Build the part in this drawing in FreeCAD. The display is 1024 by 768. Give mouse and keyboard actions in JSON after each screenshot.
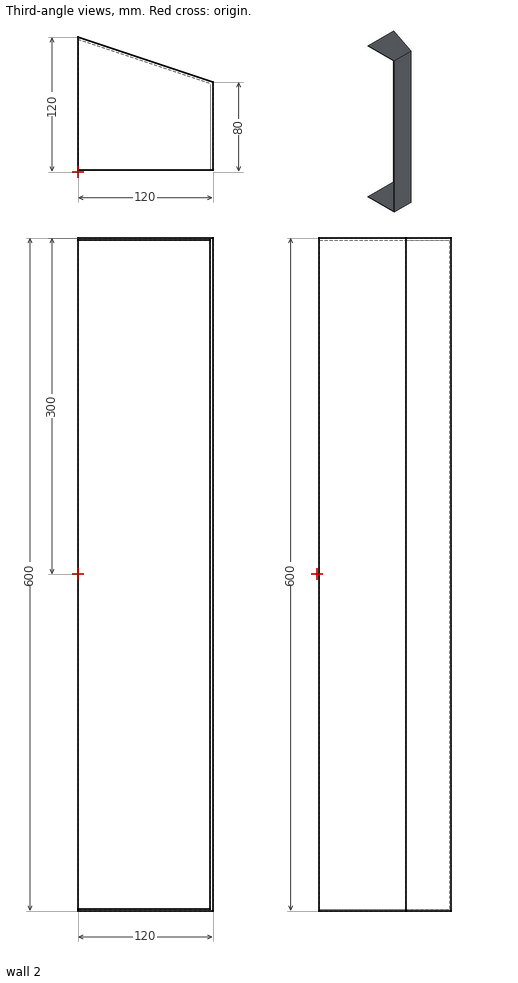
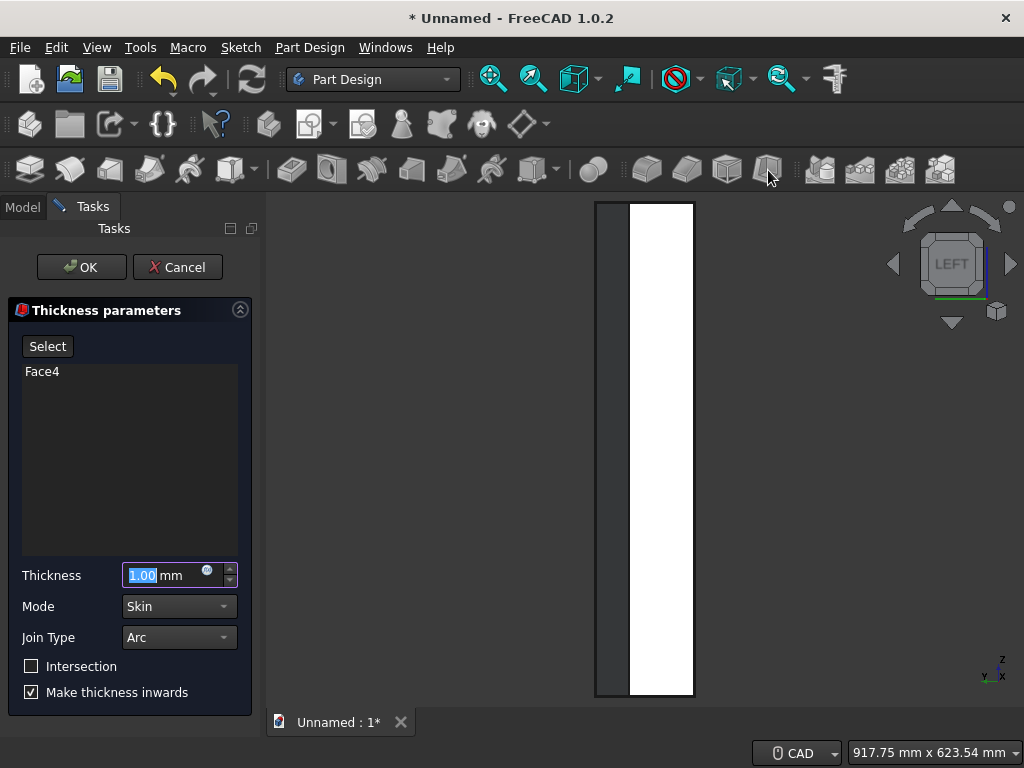
{"action": "type", "text": "2"}
{"action": "key", "text": "Tab"}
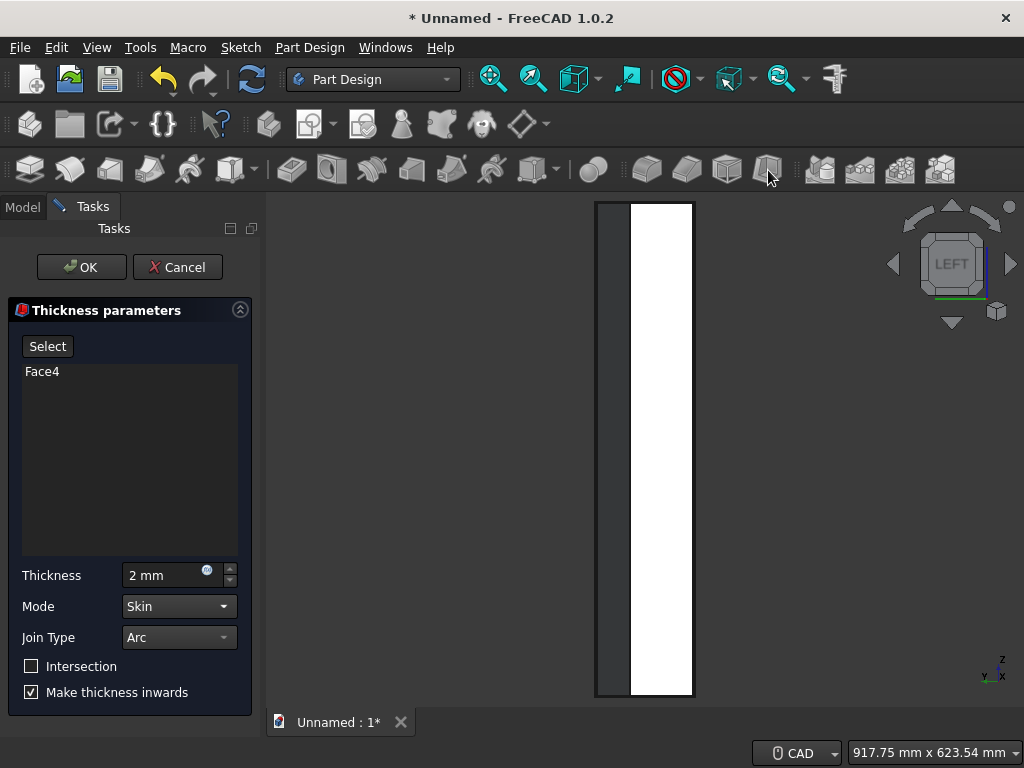
{"action": "left_click", "coordinate": [180, 638]}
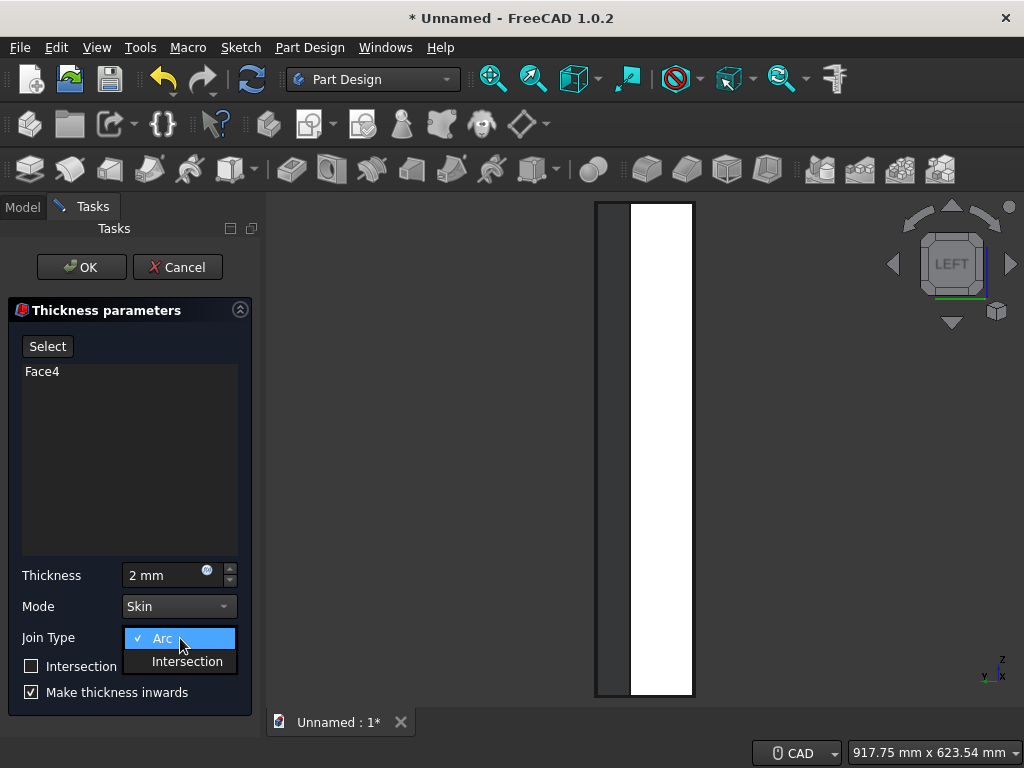
{"action": "left_click", "coordinate": [179, 662]}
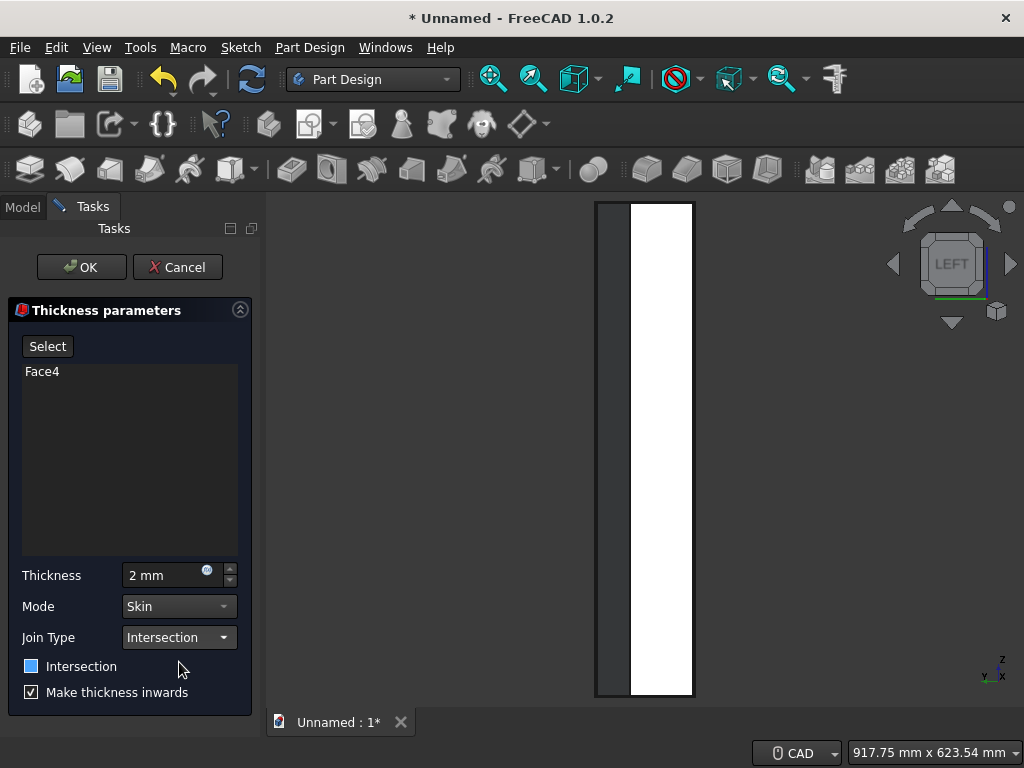
{"action": "left_click", "coordinate": [82, 267]}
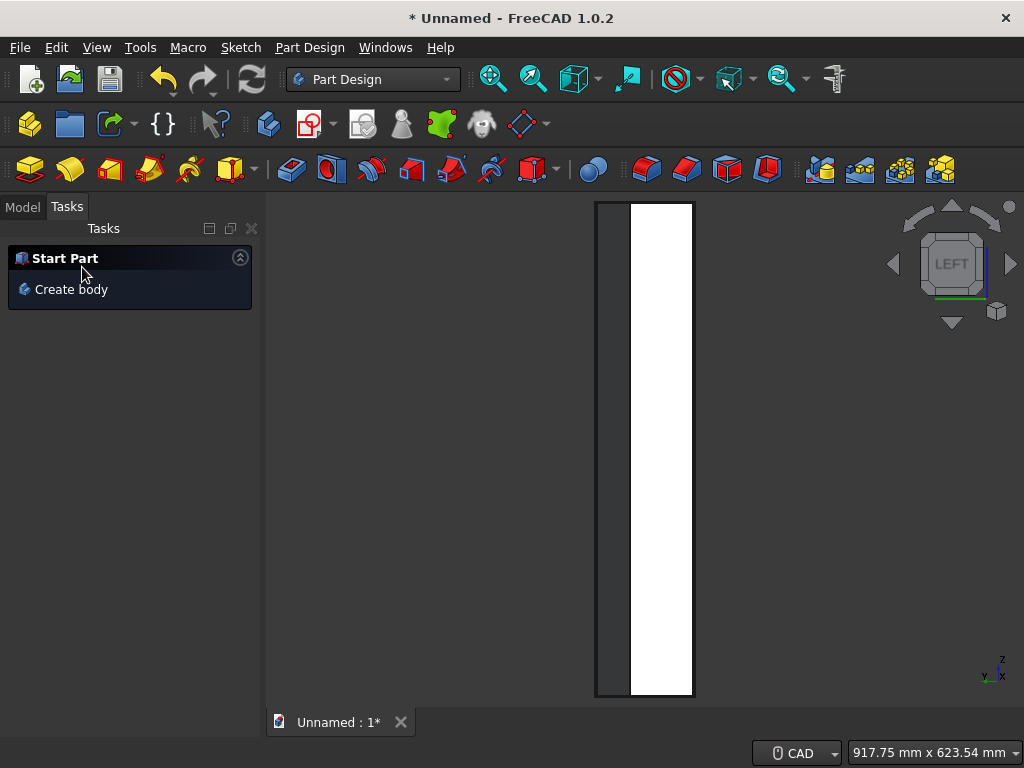
{"action": "left_click", "coordinate": [310, 124]}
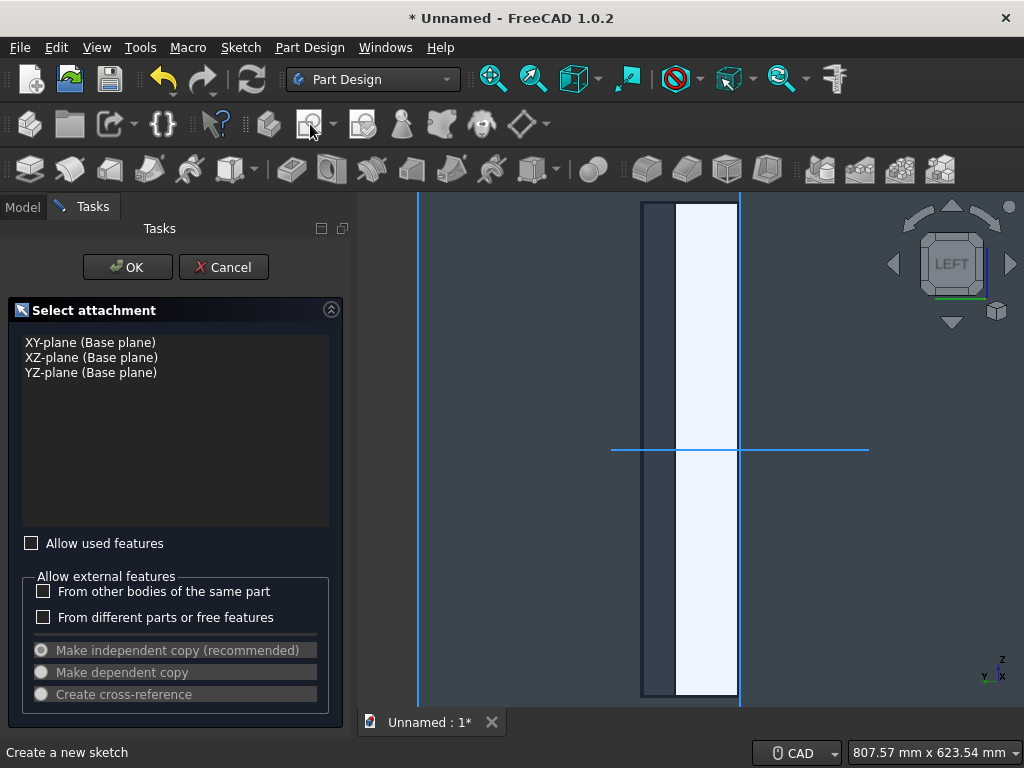
{"action": "left_click", "coordinate": [82, 358]}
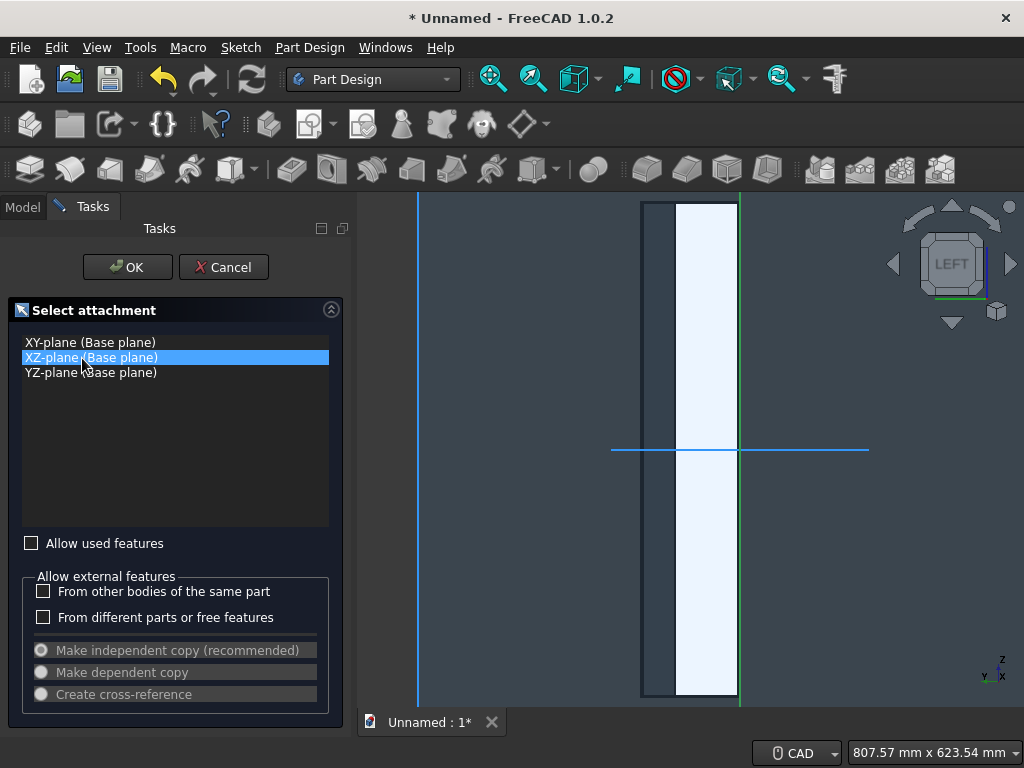
{"action": "left_click", "coordinate": [128, 267]}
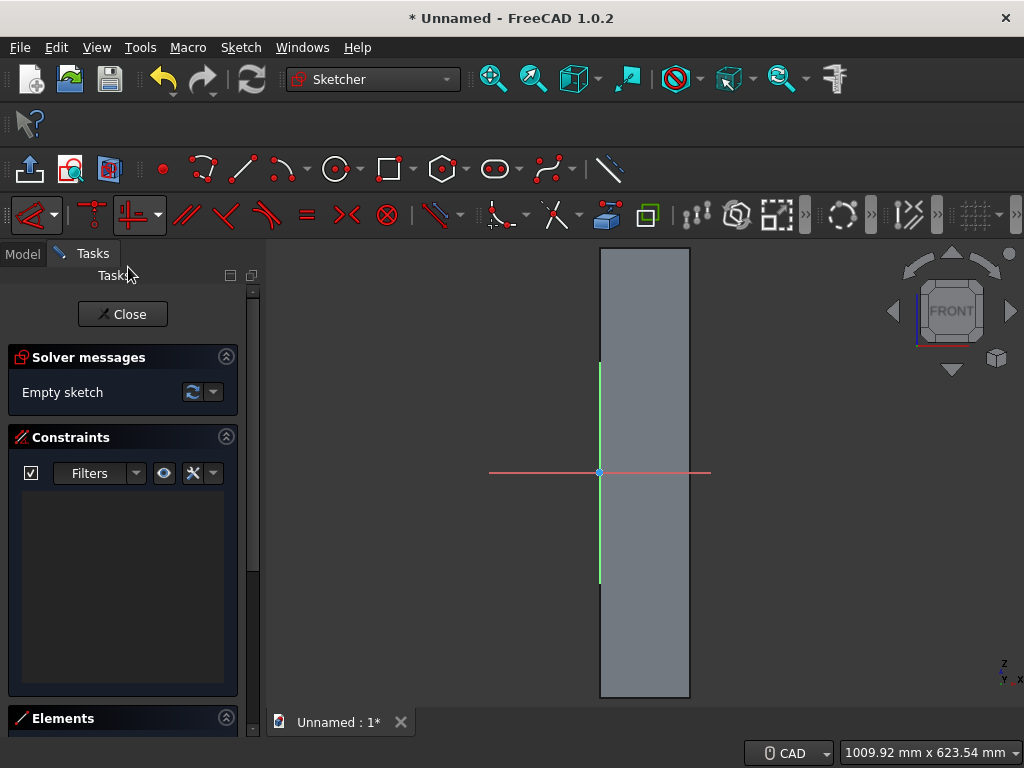
{"action": "scroll", "coordinate": [437, 473], "scroll_direction": "down", "scroll_amount": 2}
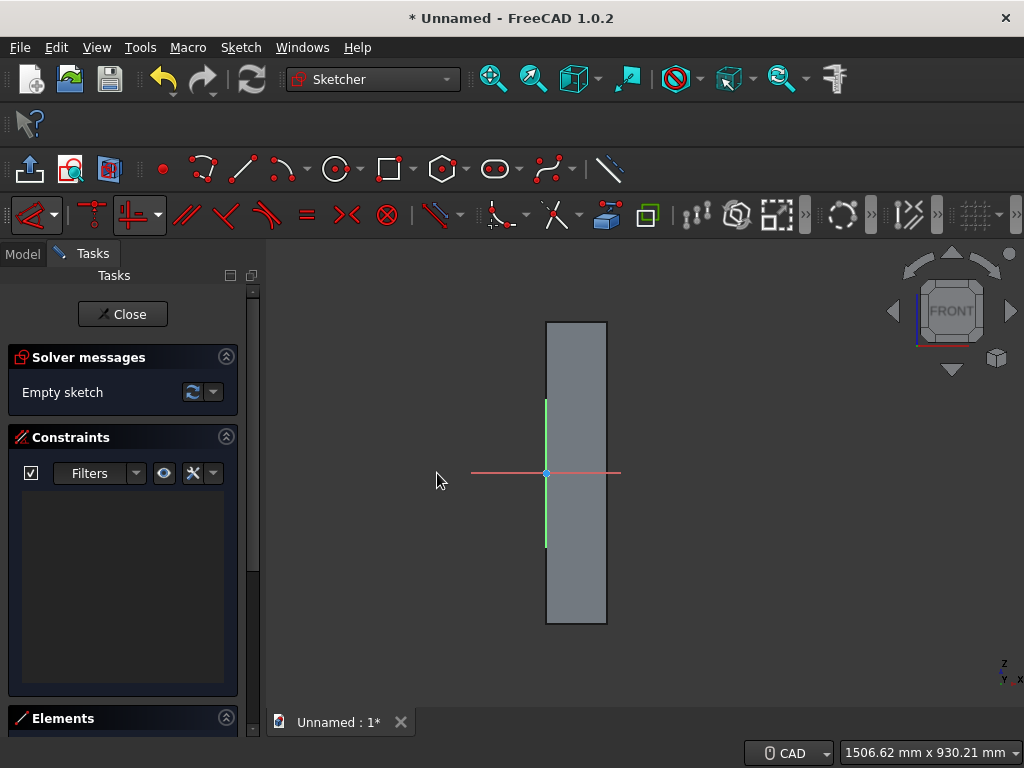
{"action": "left_click", "coordinate": [390, 170]}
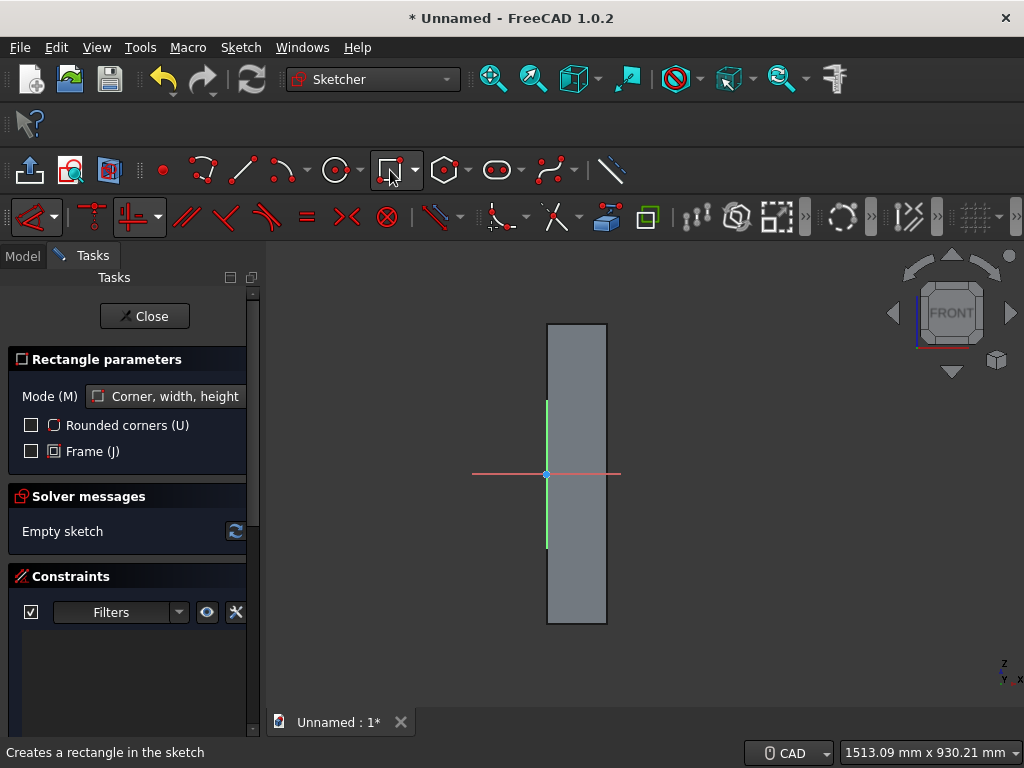
{"action": "left_click", "coordinate": [547, 324]}
{"action": "left_click", "coordinate": [607, 624]}
{"action": "key", "text": "Escape"}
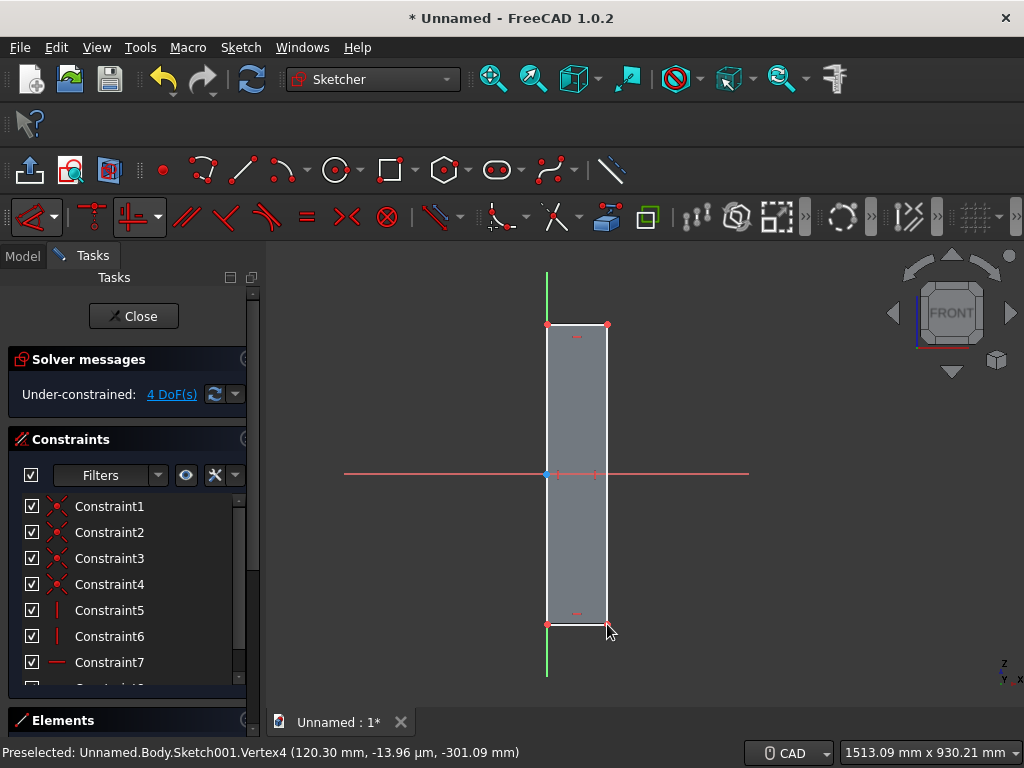
{"action": "left_click", "coordinate": [547, 325]}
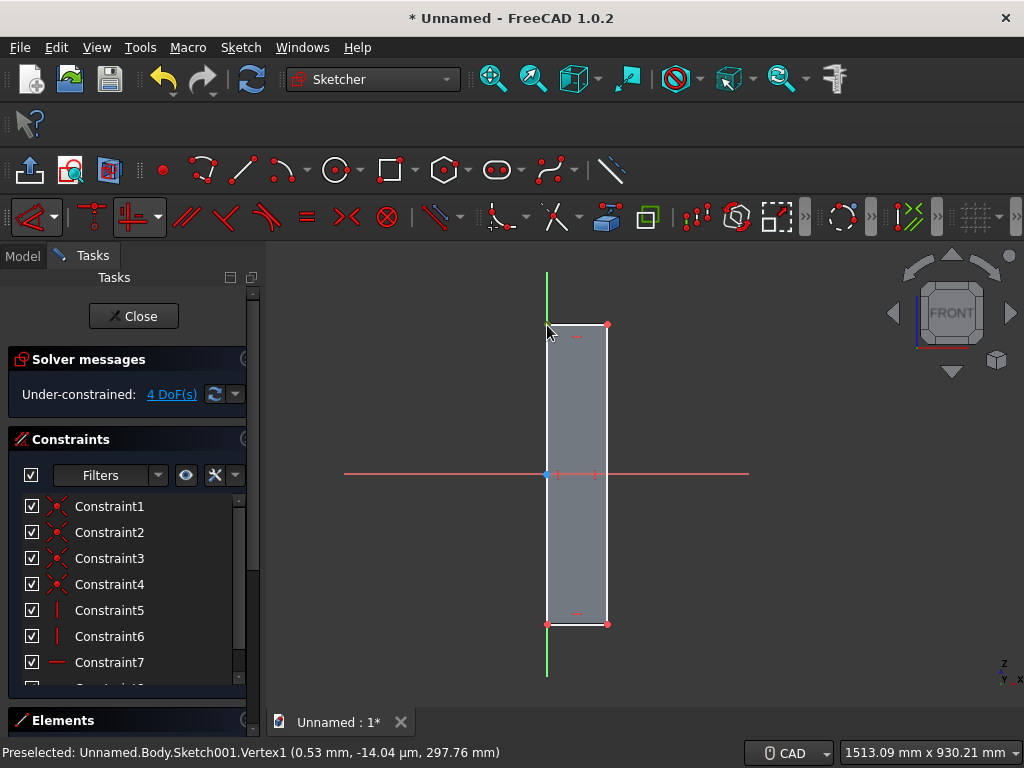
{"action": "left_click", "coordinate": [547, 298]}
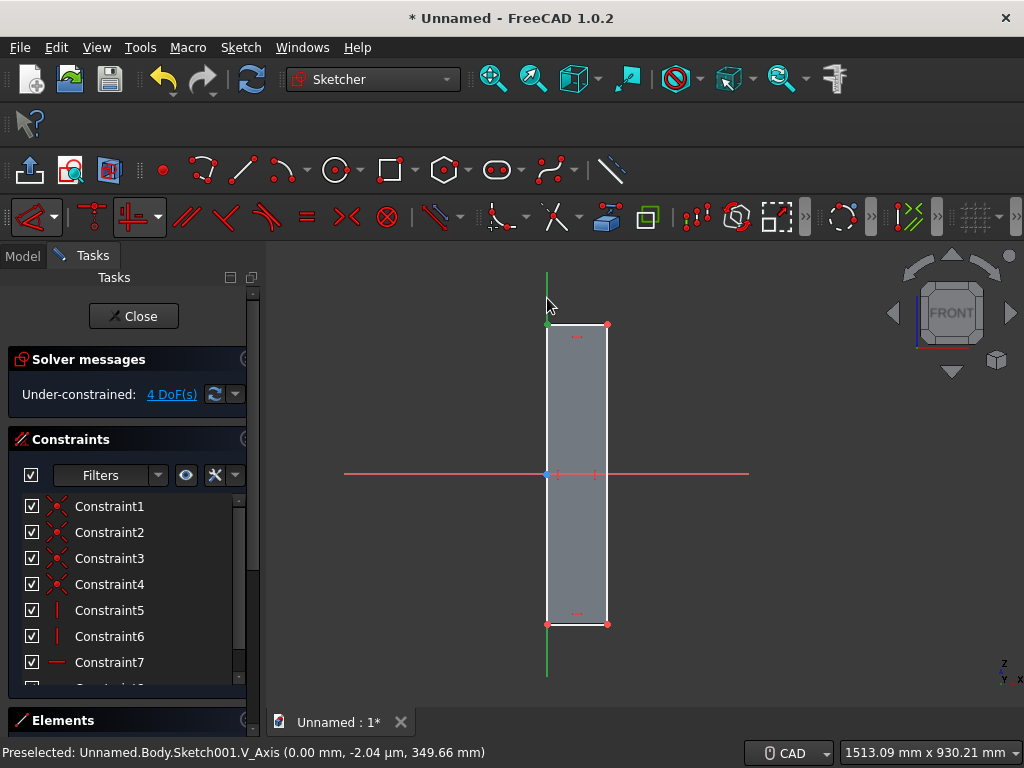
{"action": "left_click", "coordinate": [92, 218]}